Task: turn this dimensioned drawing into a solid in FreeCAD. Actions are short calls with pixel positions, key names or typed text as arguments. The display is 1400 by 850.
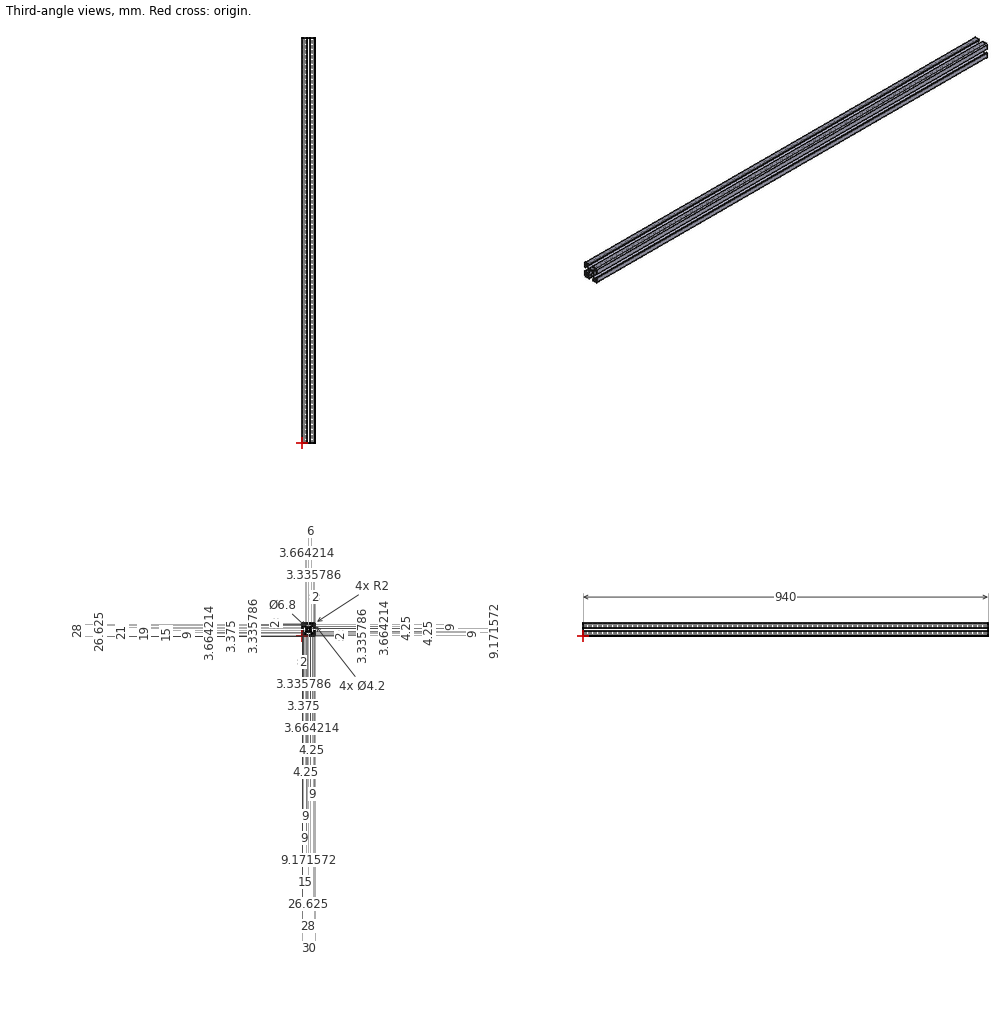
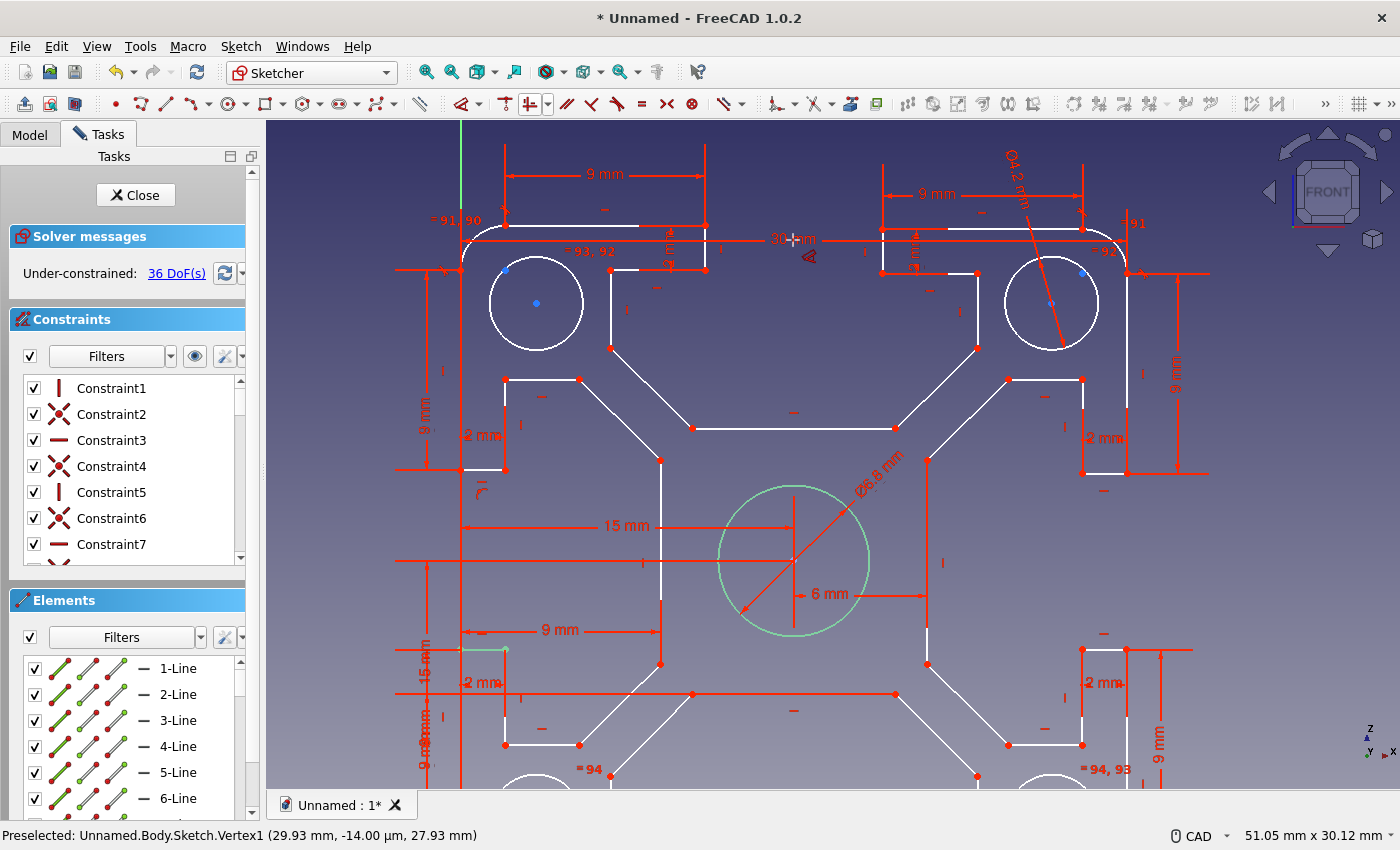
click(1127, 274)
click(1161, 517)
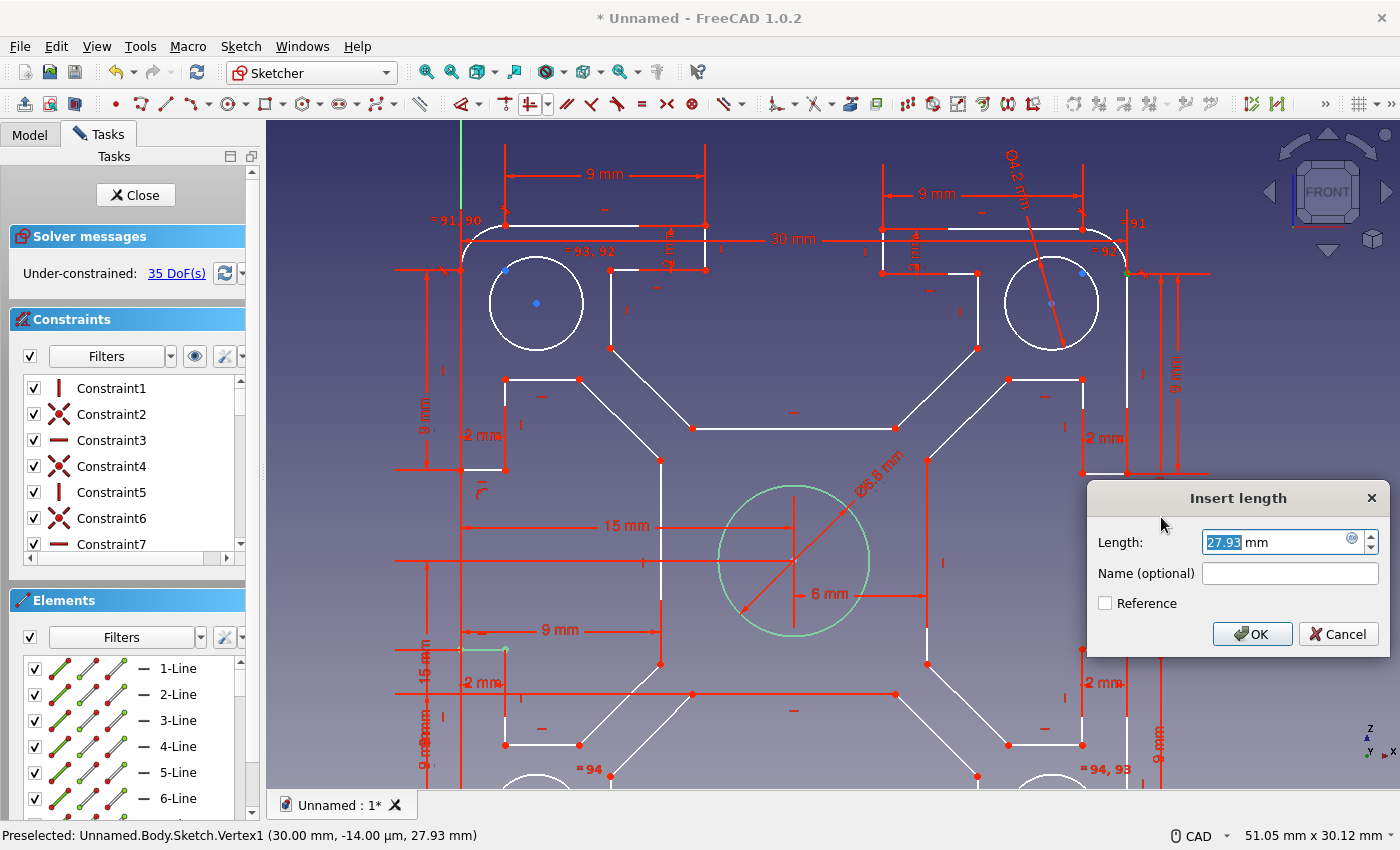
text(28)
key(Return)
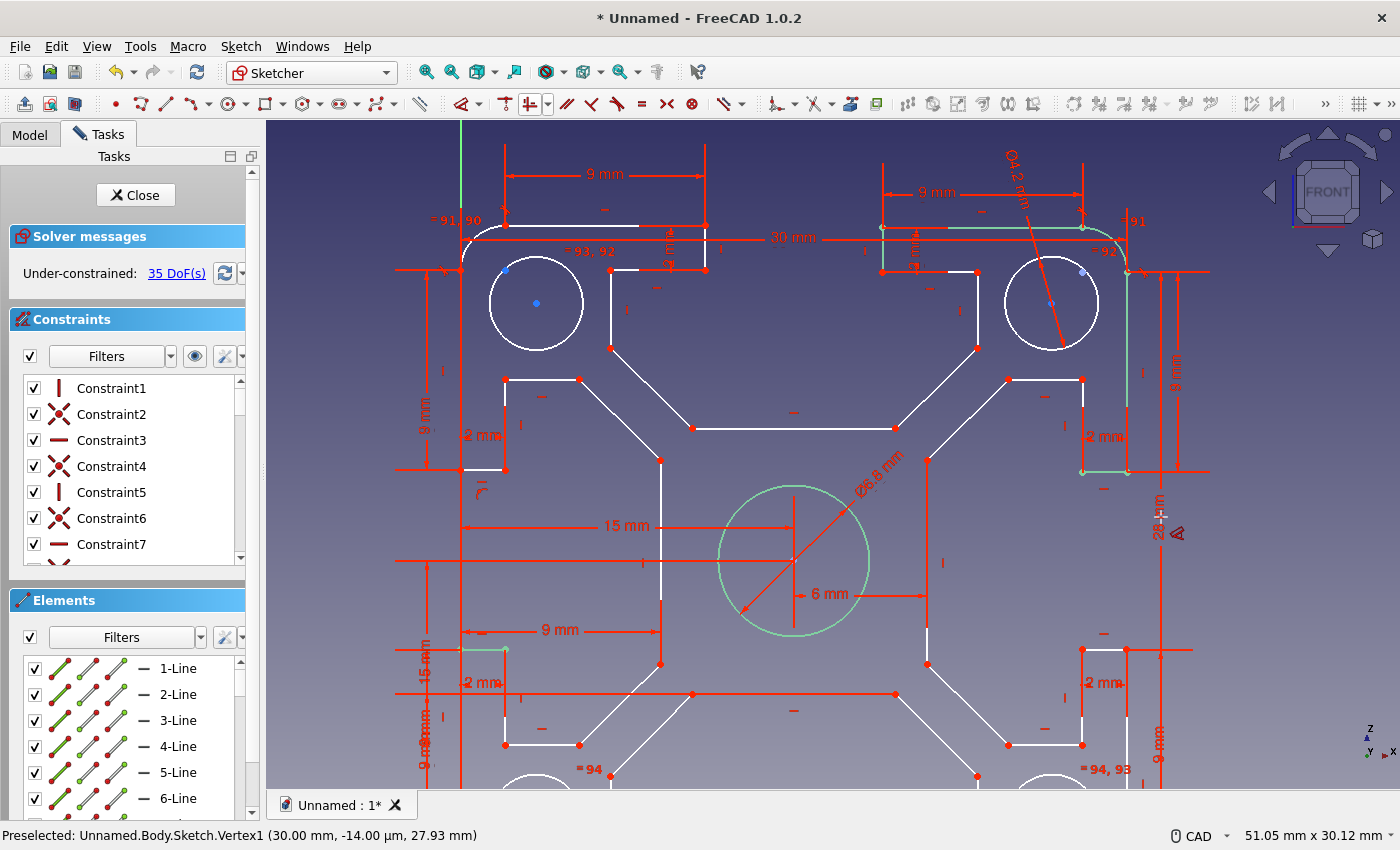
click(1082, 745)
click(771, 711)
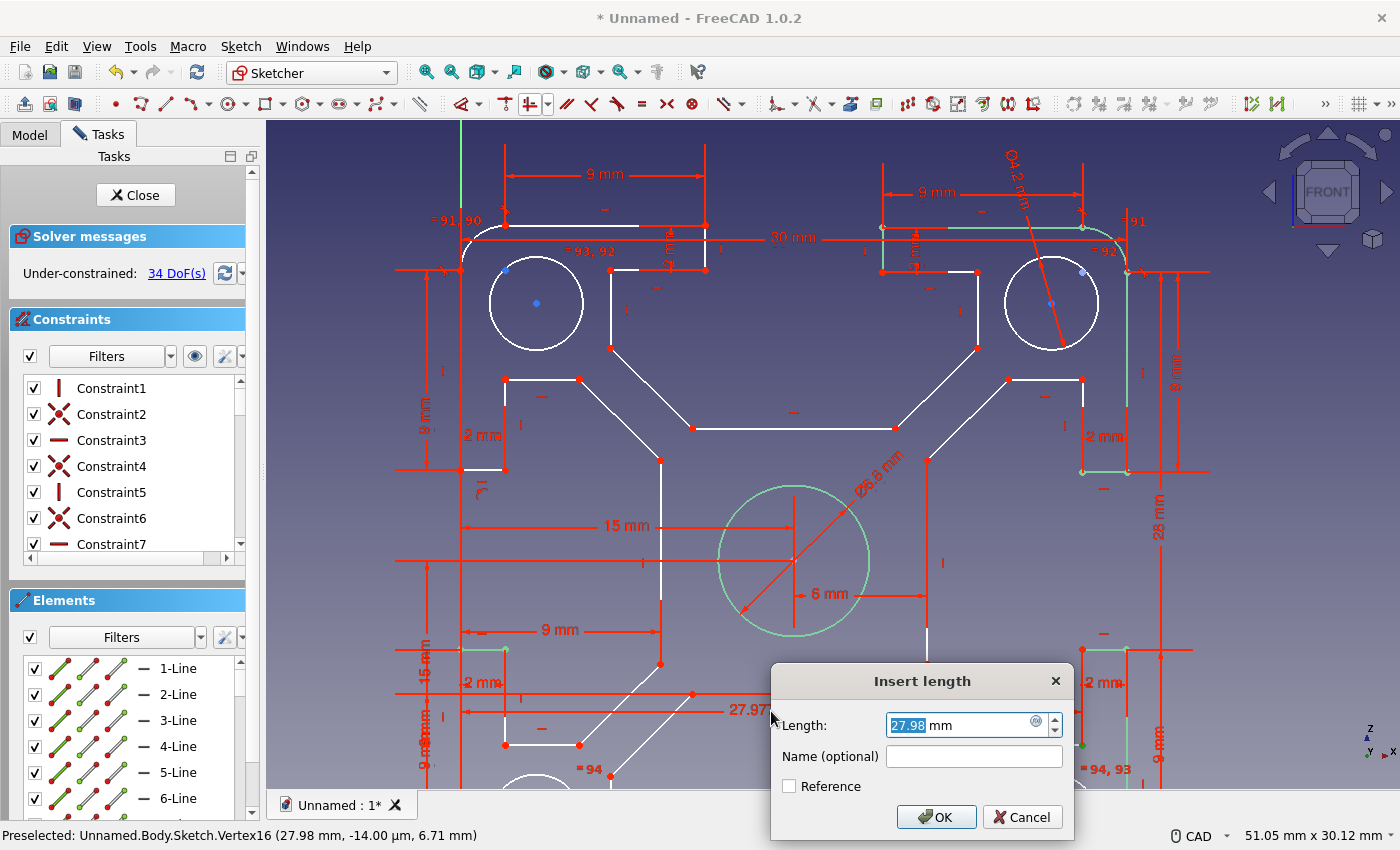
text(28)
key(Return)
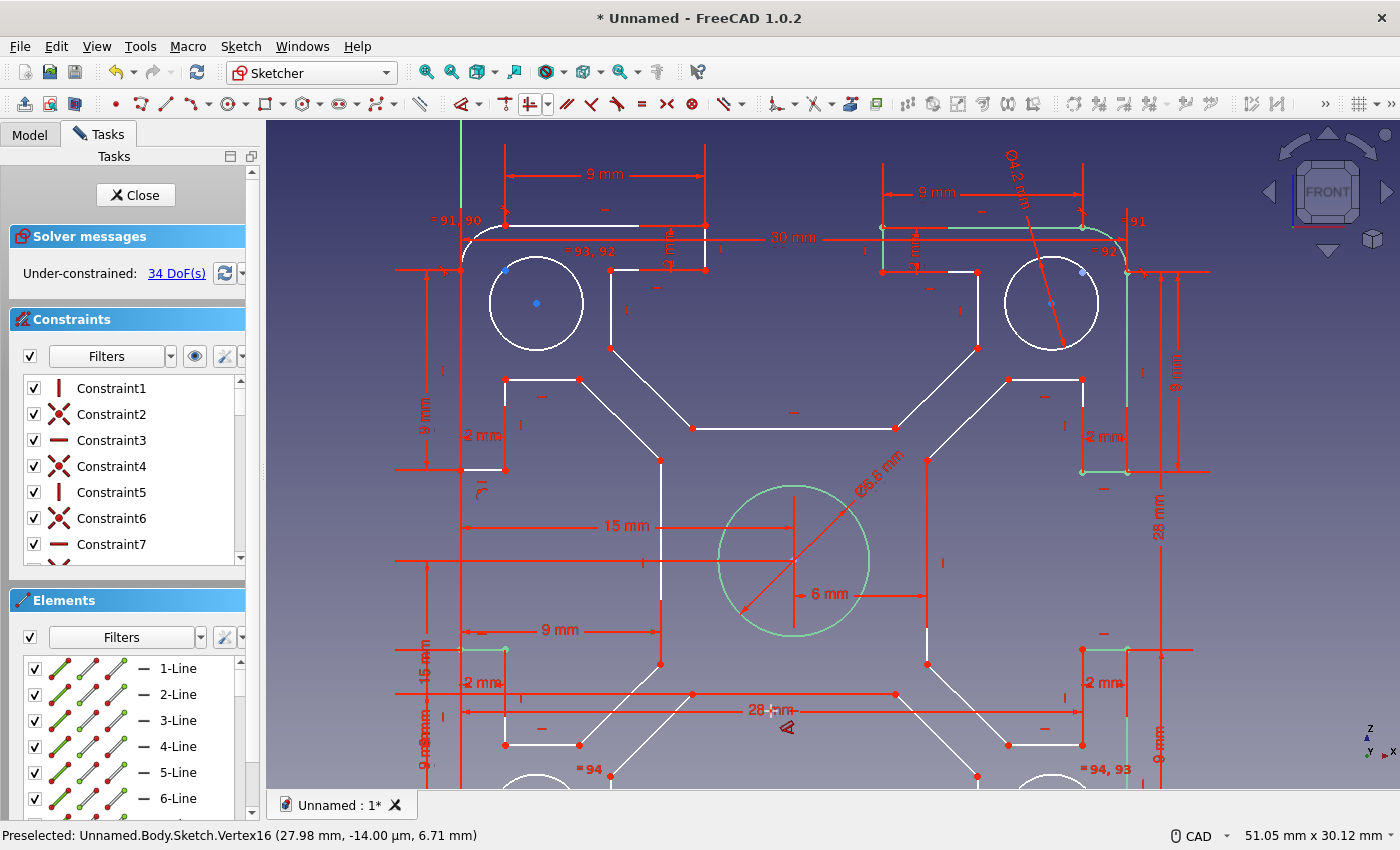
click(505, 470)
click(427, 616)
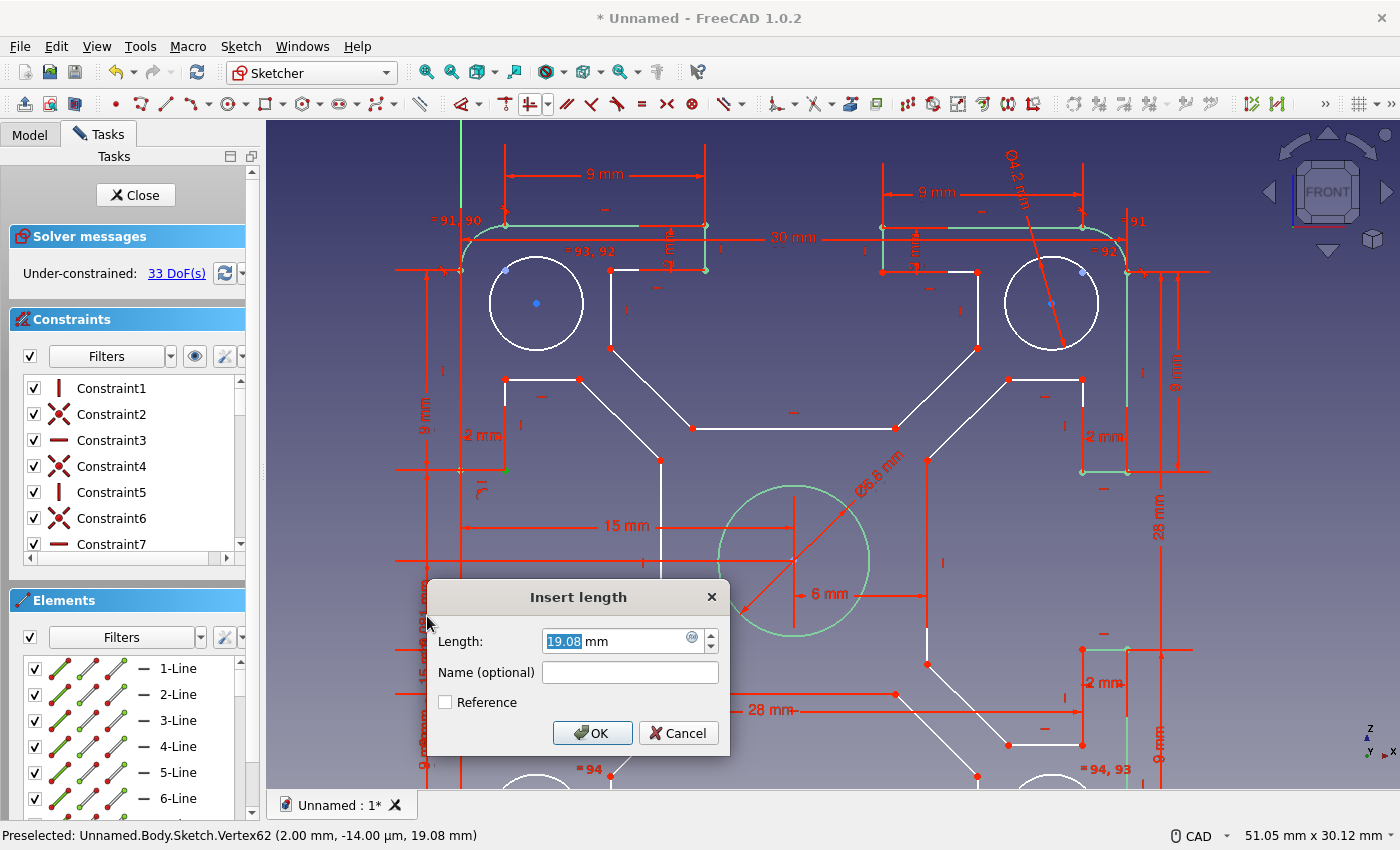
text(19)
key(Return)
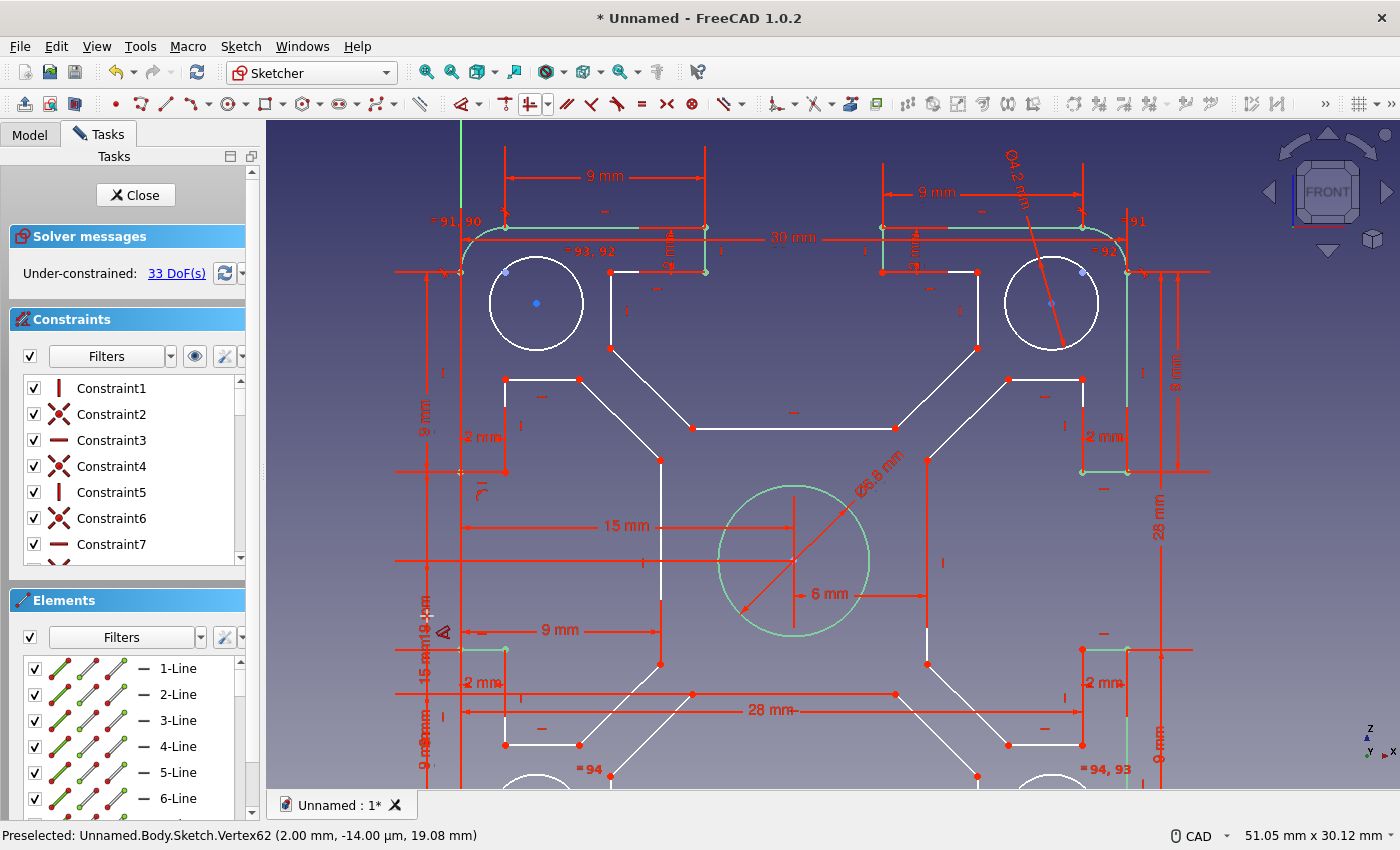
click(693, 429)
click(427, 595)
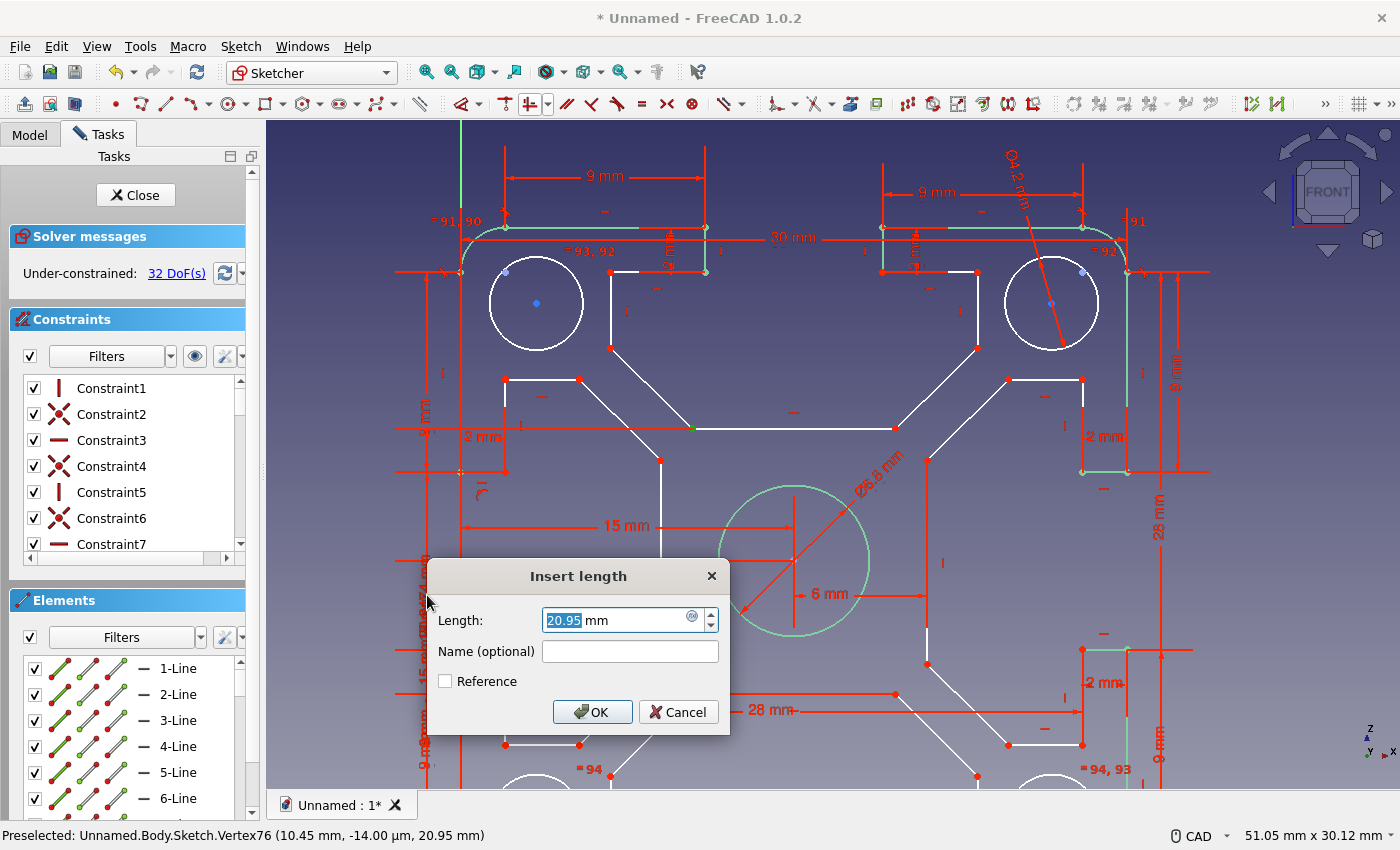
text(21)
key(Return)